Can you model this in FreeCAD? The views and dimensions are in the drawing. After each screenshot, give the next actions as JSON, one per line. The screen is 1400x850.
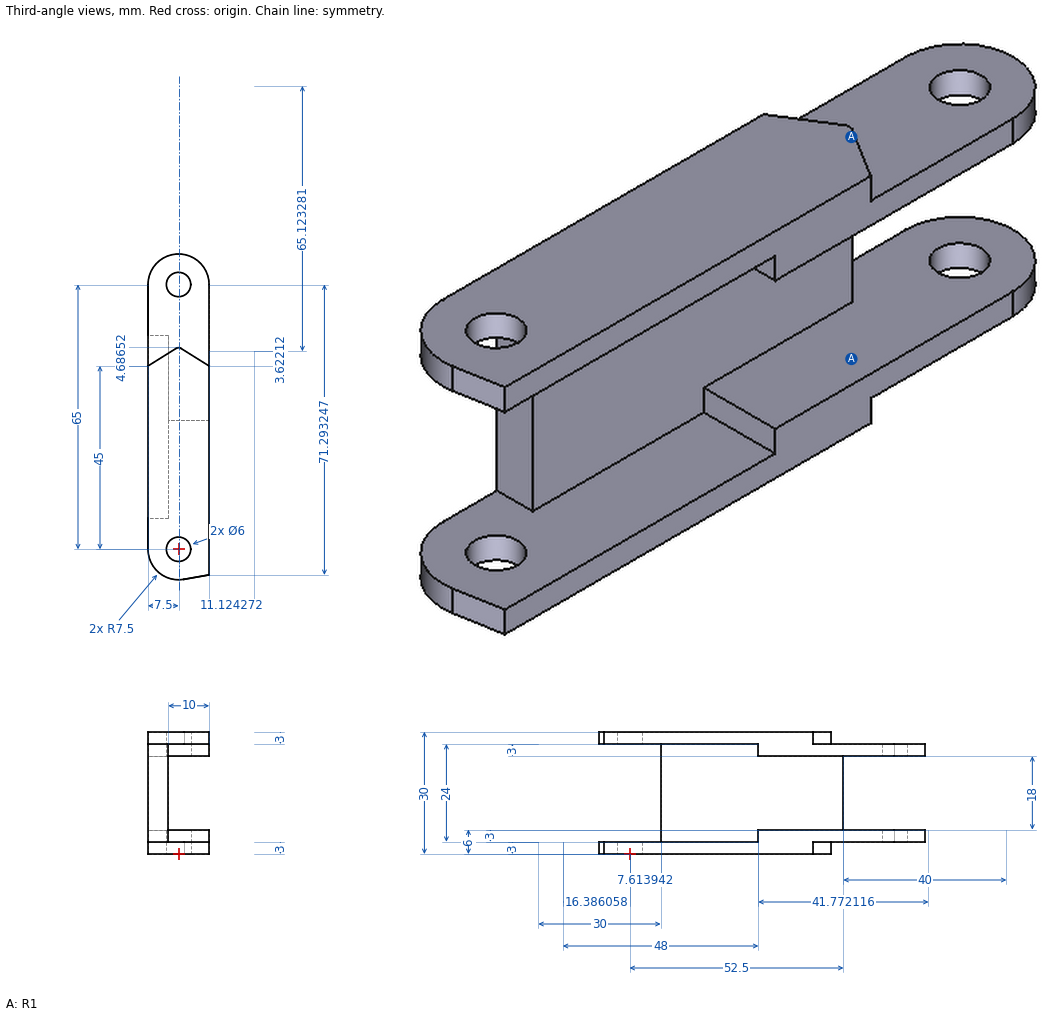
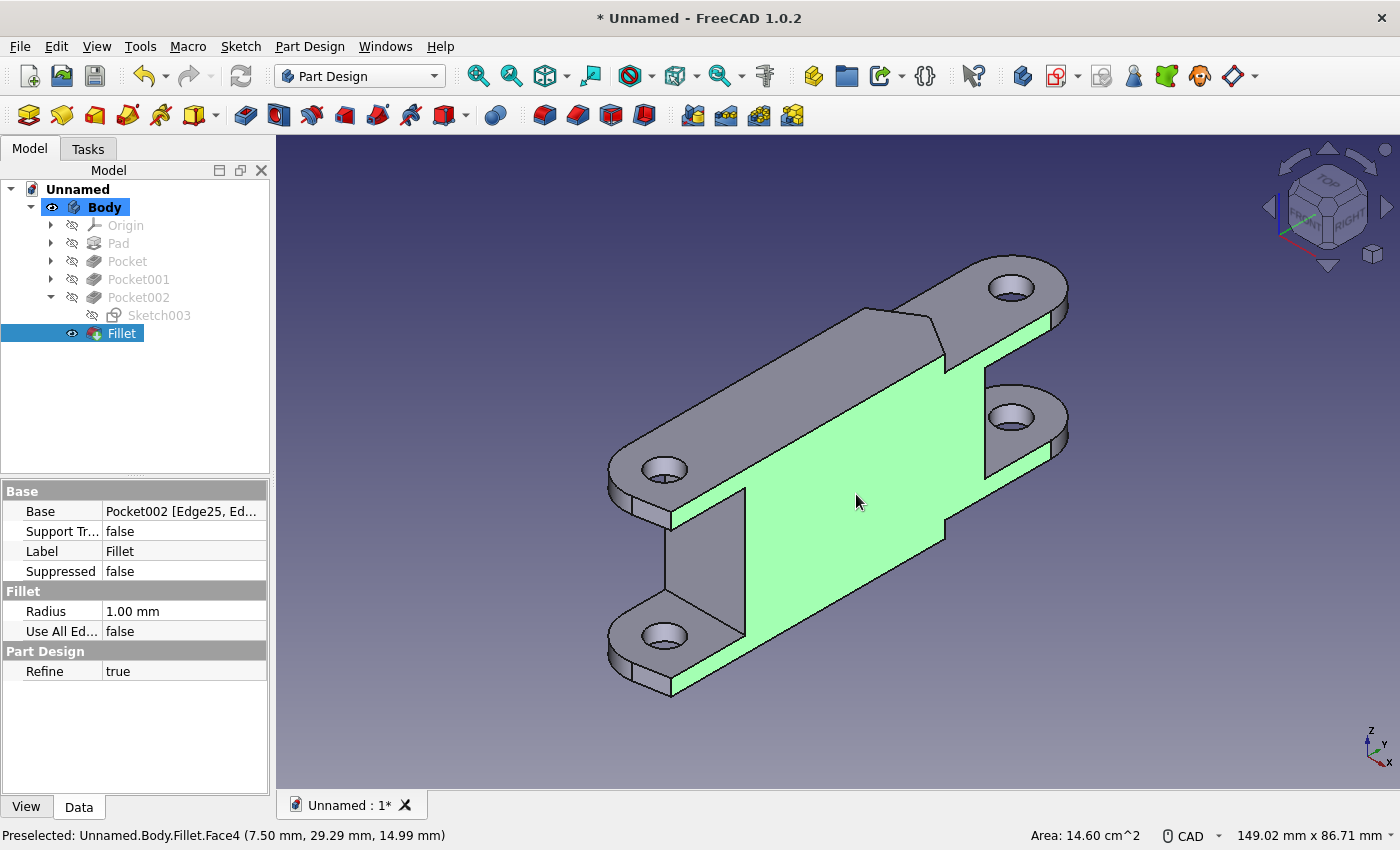
{"action": "left_click", "coordinate": [1056, 76]}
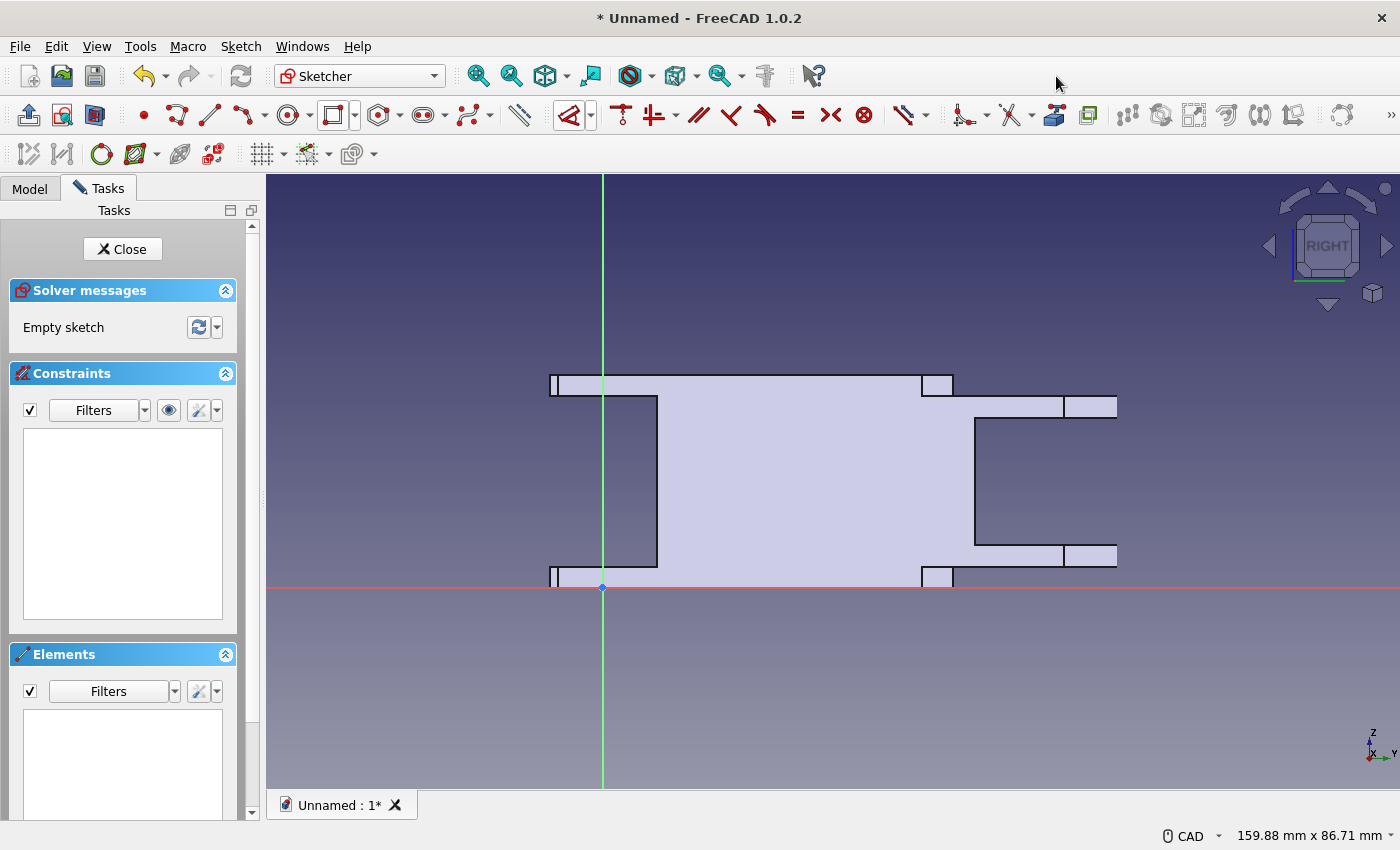
{"action": "key", "text": "g m"}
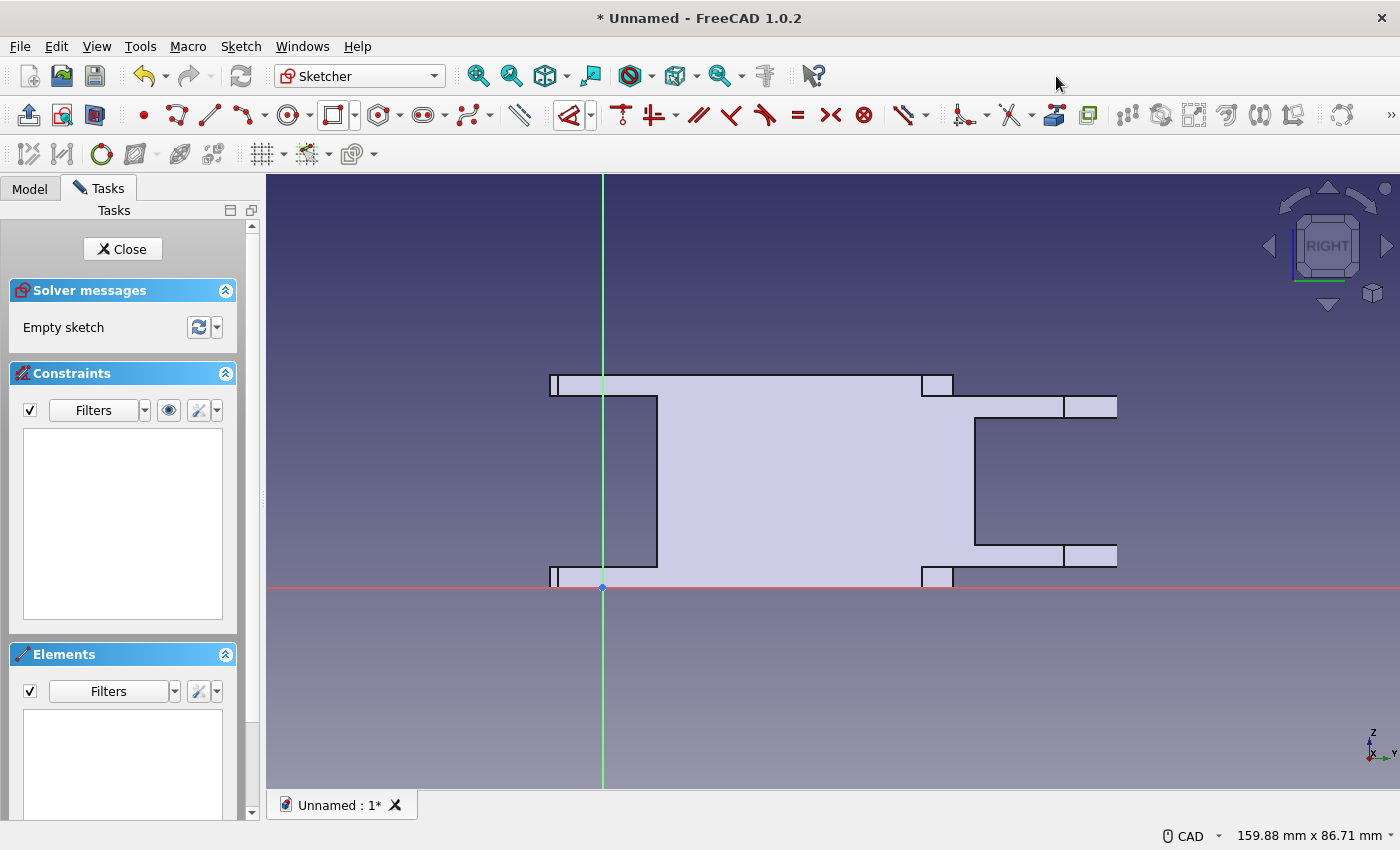
{"action": "left_click", "coordinate": [486, 567]}
{"action": "left_click", "coordinate": [827, 567]}
{"action": "left_click", "coordinate": [827, 545]}
{"action": "left_click", "coordinate": [1123, 545]}
{"action": "left_click", "coordinate": [1123, 418]}
{"action": "left_click", "coordinate": [827, 418]}
{"action": "left_click", "coordinate": [827, 396]}
{"action": "left_click", "coordinate": [486, 396]}
{"action": "left_click", "coordinate": [486, 568]}
{"action": "key", "text": "Escape"}
{"action": "key", "text": "Escape"}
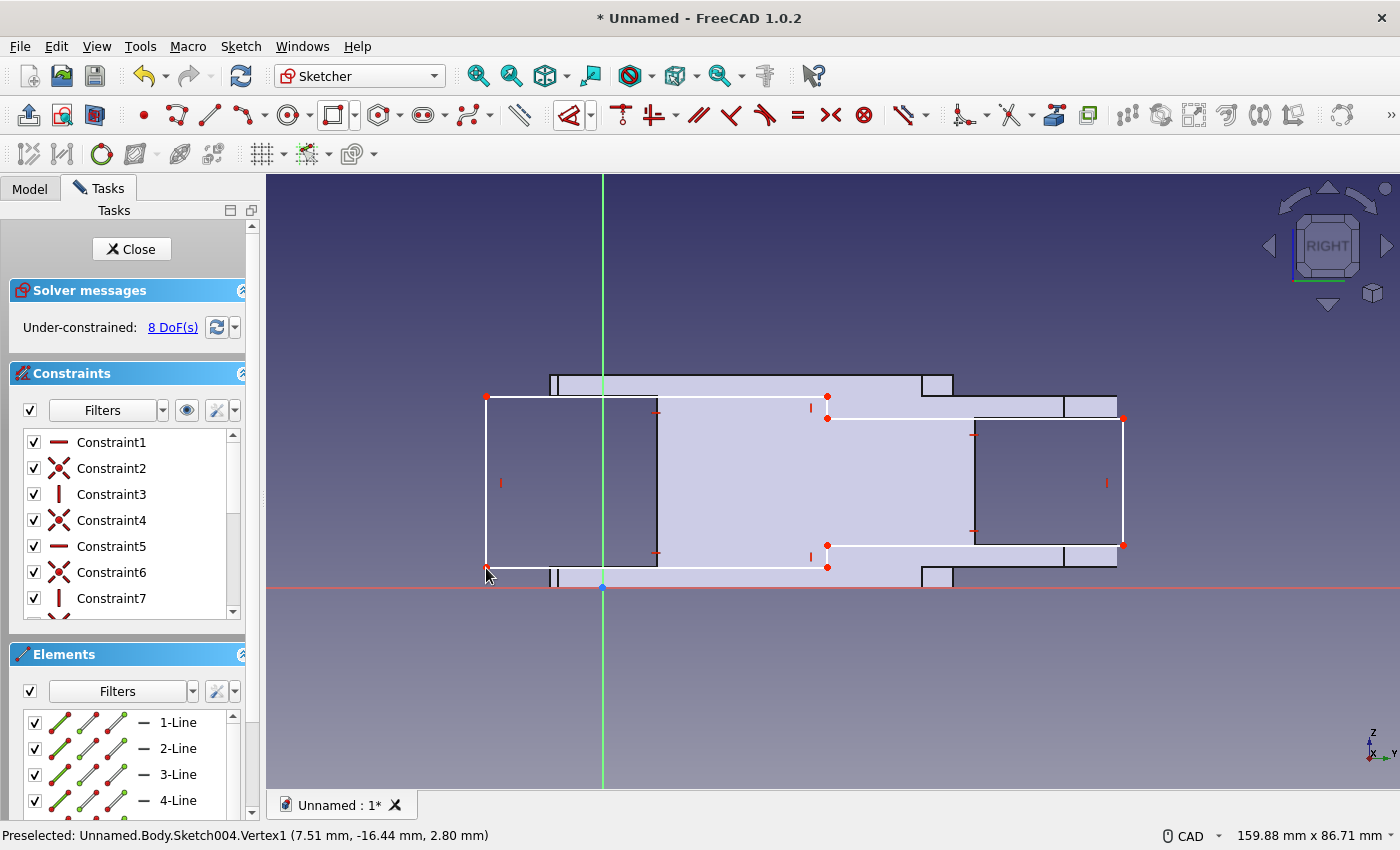
{"action": "scroll", "coordinate": [827, 557], "scroll_direction": "up", "scroll_amount": 4}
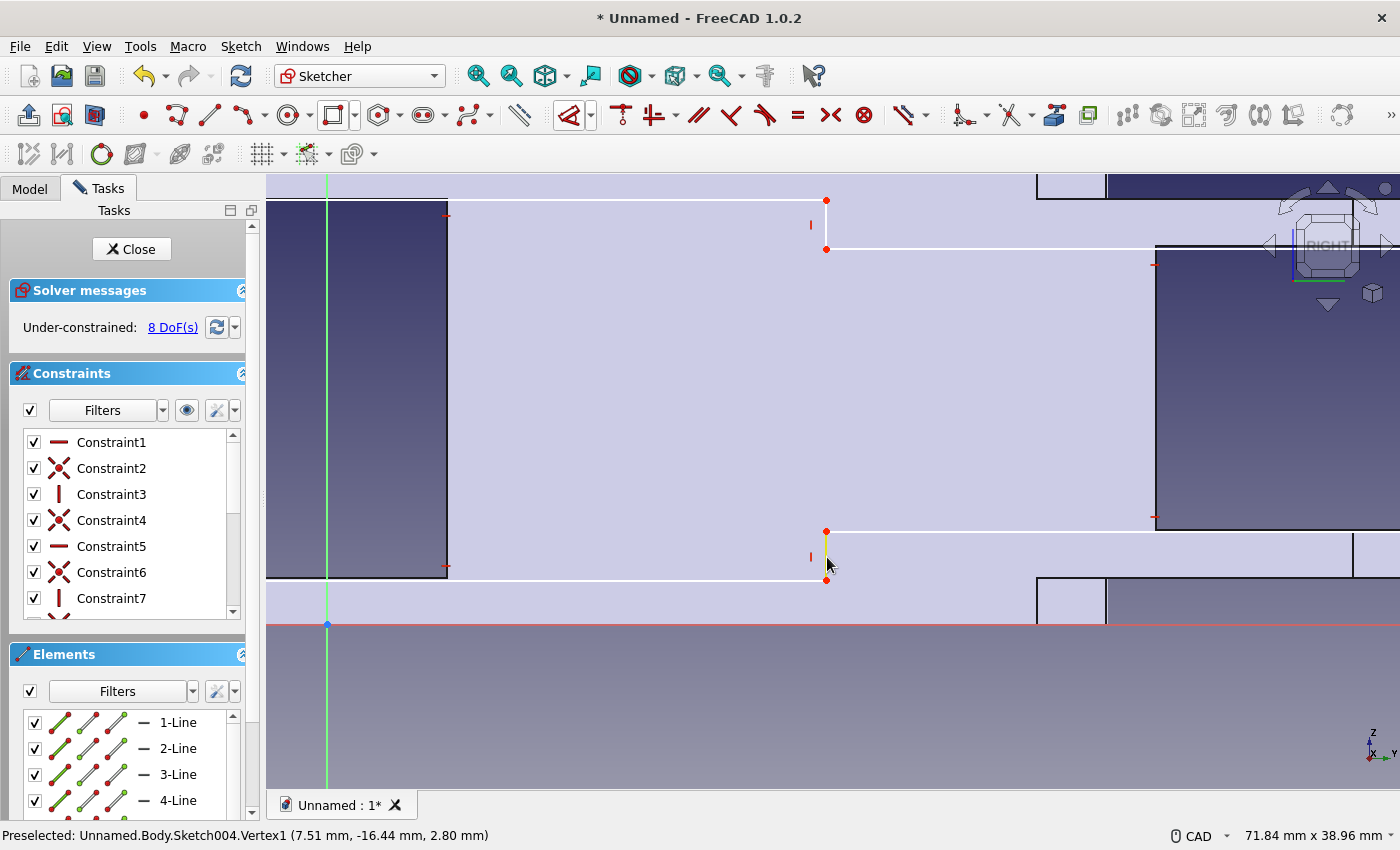
{"action": "left_click", "coordinate": [826, 556]}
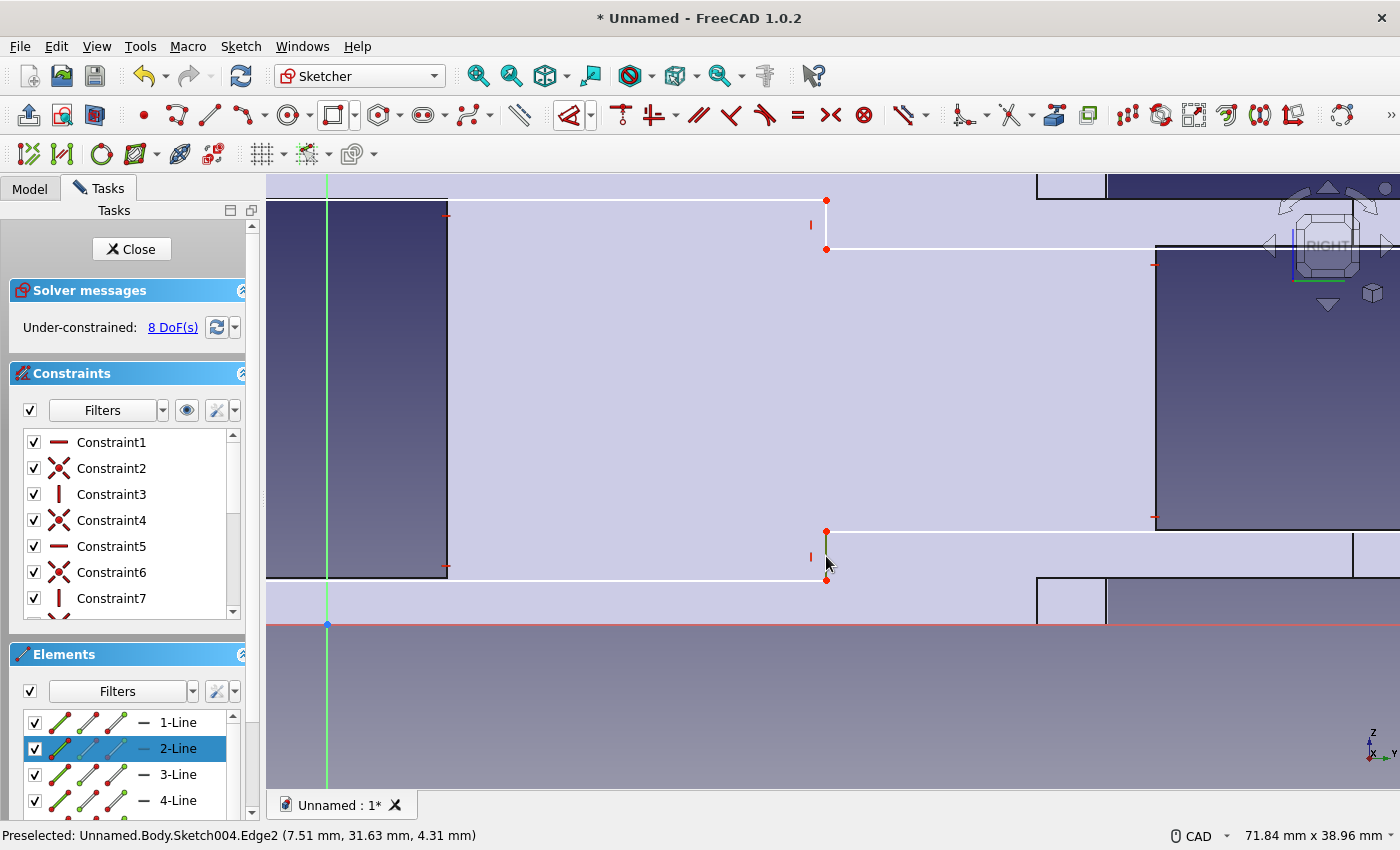
{"action": "key", "text": "i"}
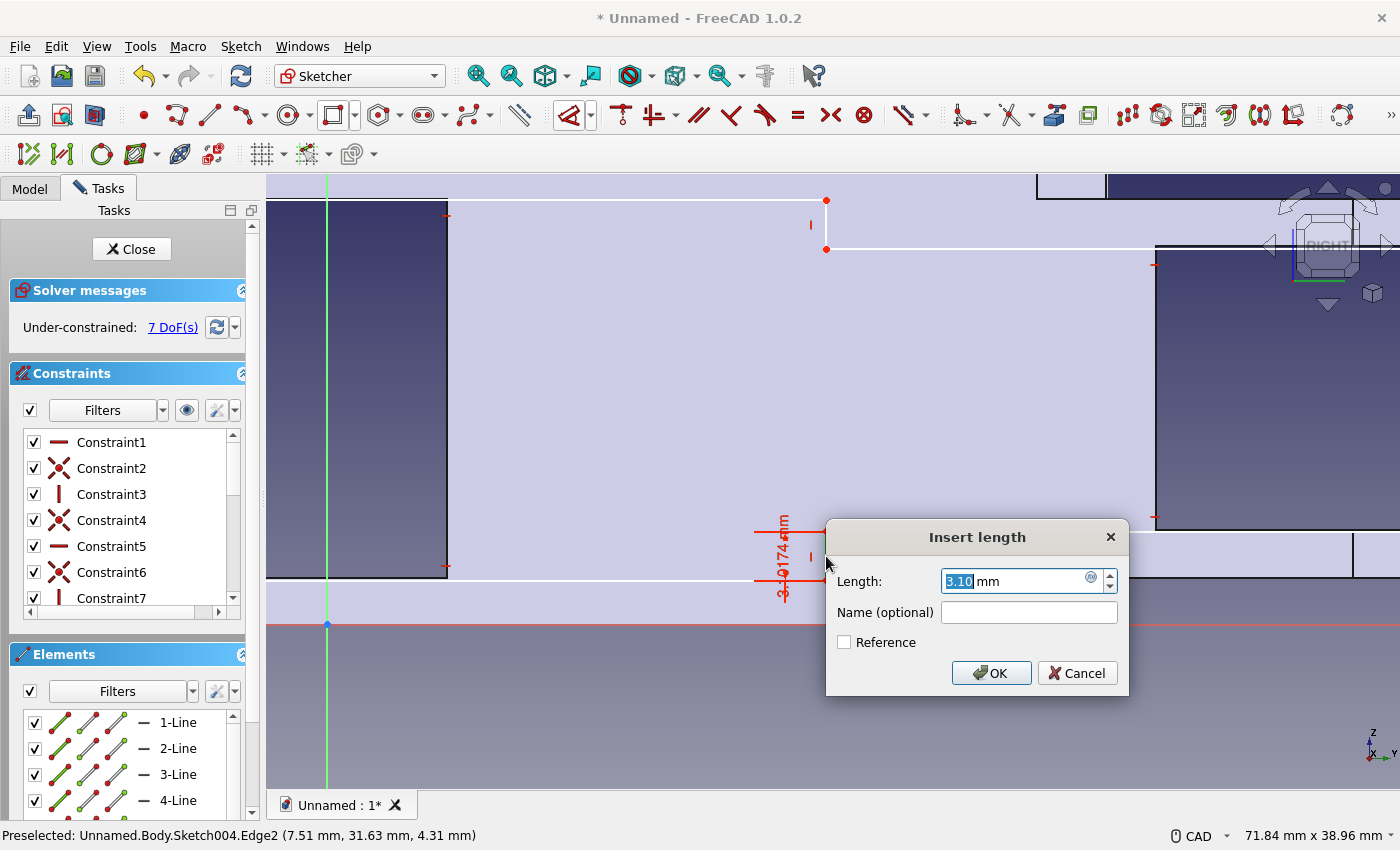
{"action": "type", "text": "3"}
{"action": "key", "text": "Return"}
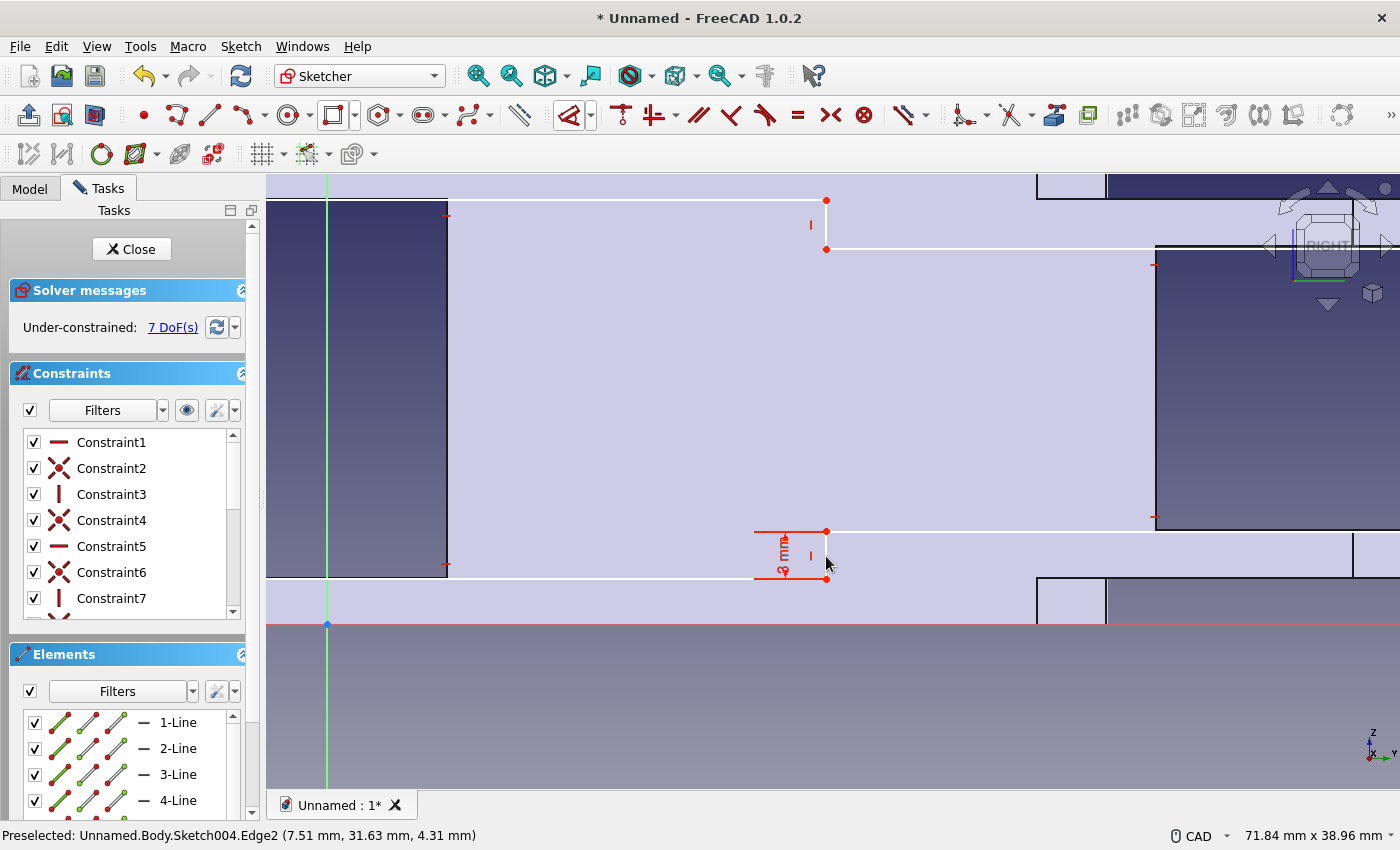
{"action": "left_click", "coordinate": [826, 234]}